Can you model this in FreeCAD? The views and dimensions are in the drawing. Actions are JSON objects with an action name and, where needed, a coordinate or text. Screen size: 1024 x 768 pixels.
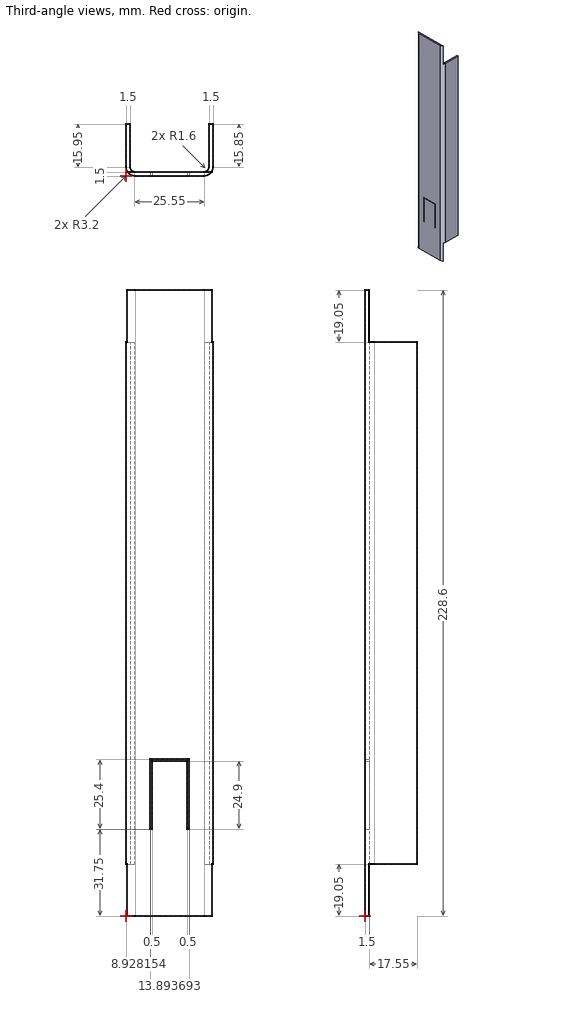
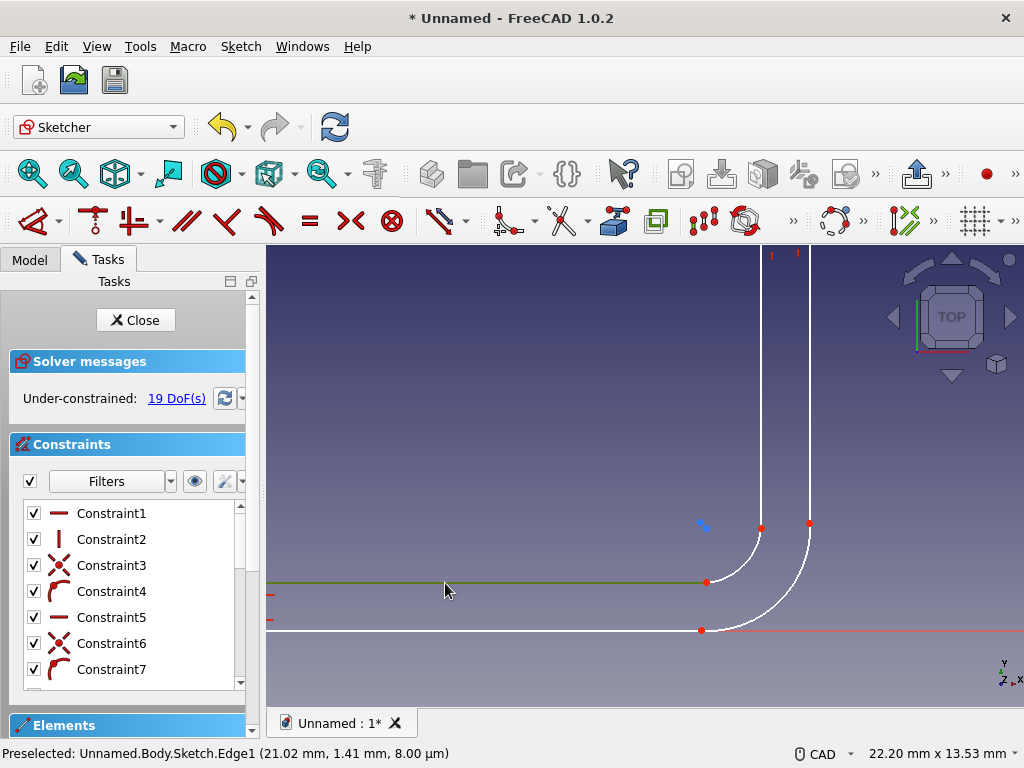
{"action": "scroll", "coordinate": [755, 575], "scroll_direction": "down", "scroll_amount": 5}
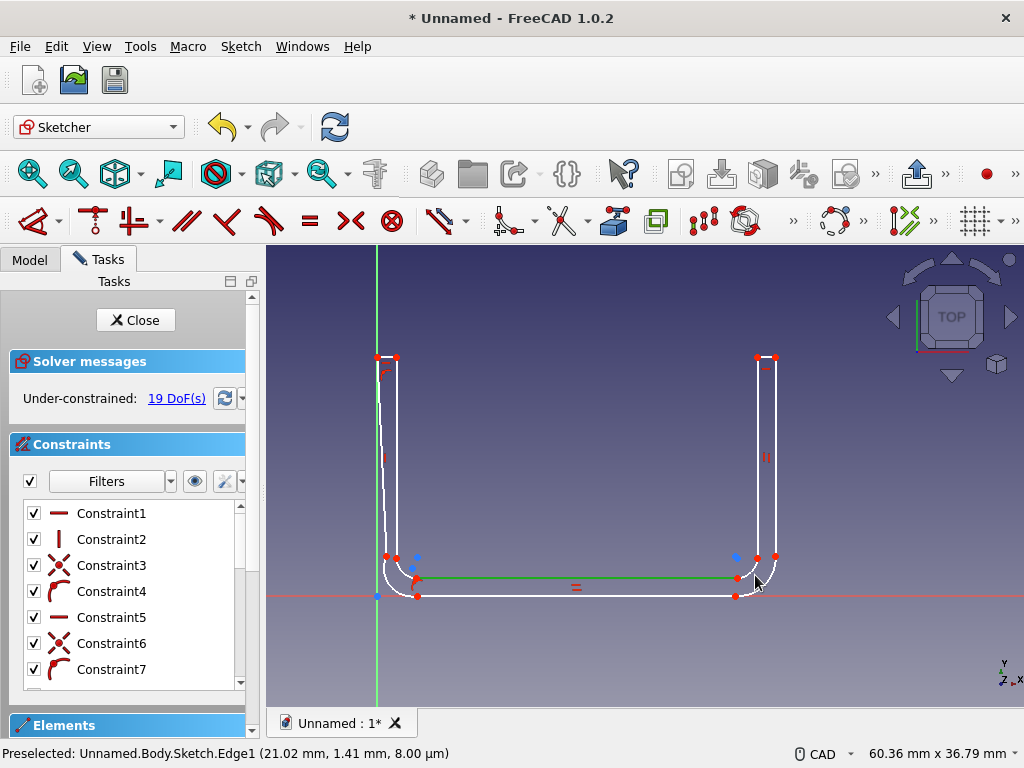
{"action": "scroll", "coordinate": [399, 567], "scroll_direction": "up", "scroll_amount": 2}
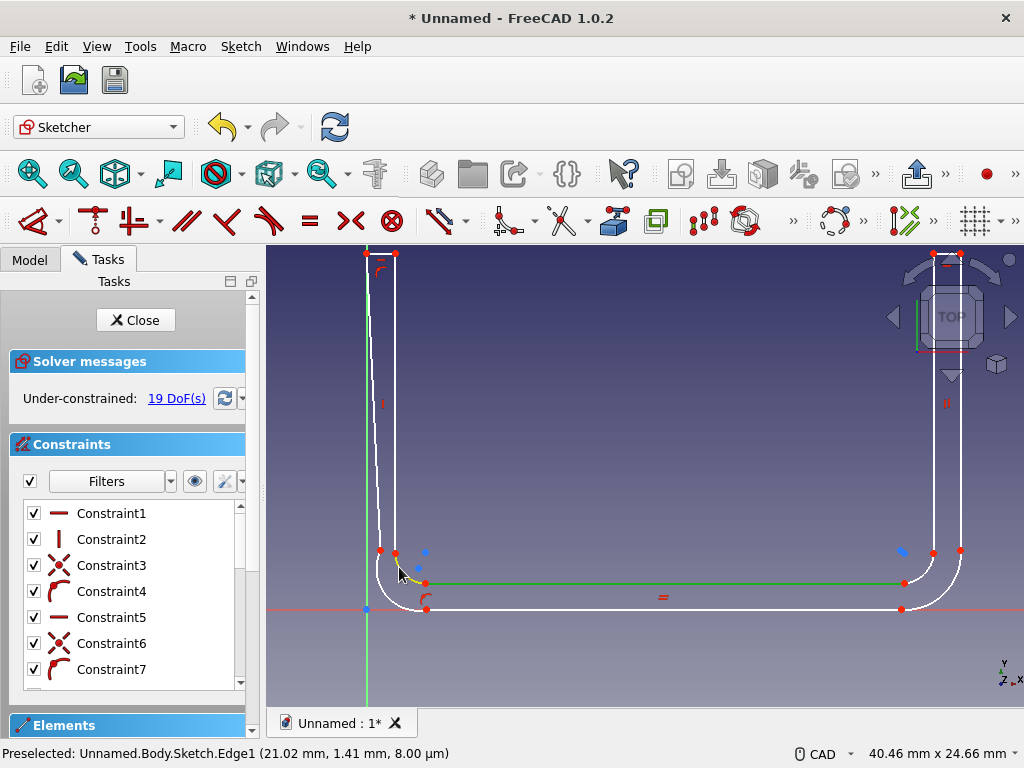
{"action": "left_click", "coordinate": [399, 567]}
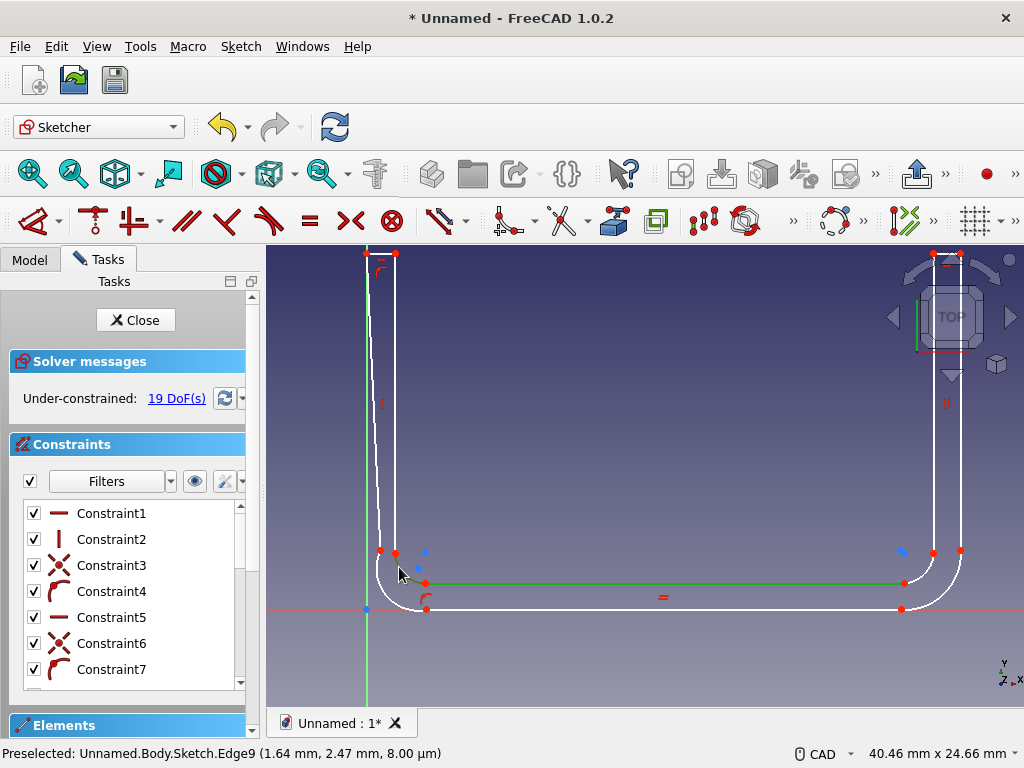
{"action": "left_click", "coordinate": [269, 222]}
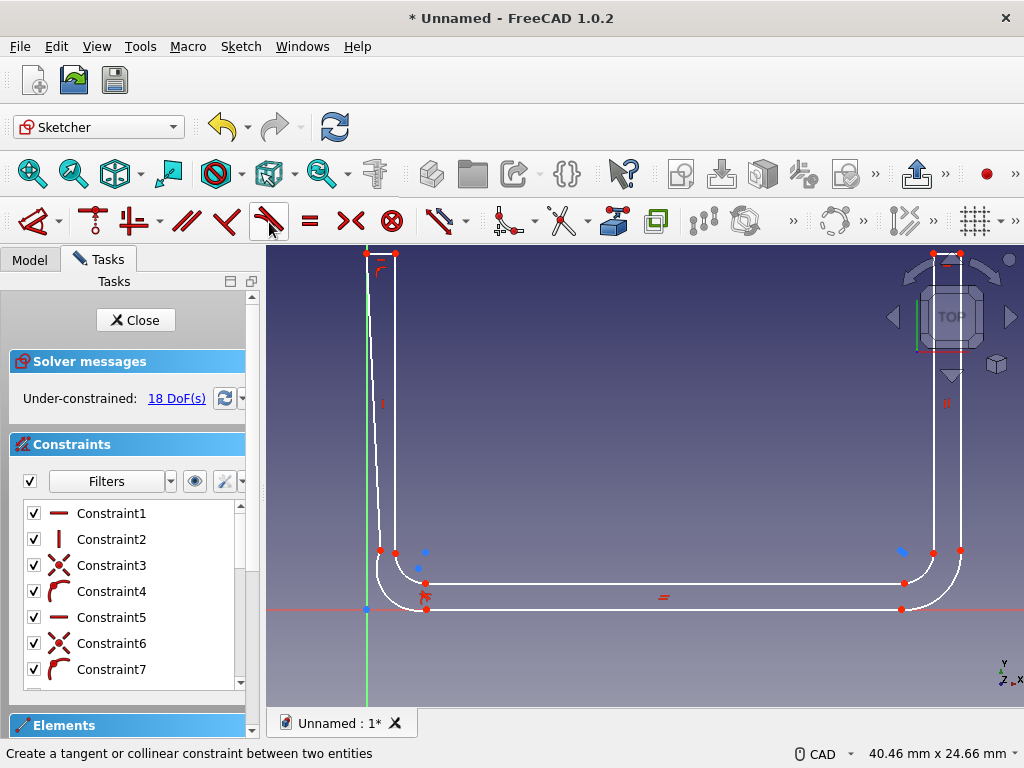
{"action": "left_click", "coordinate": [761, 584]}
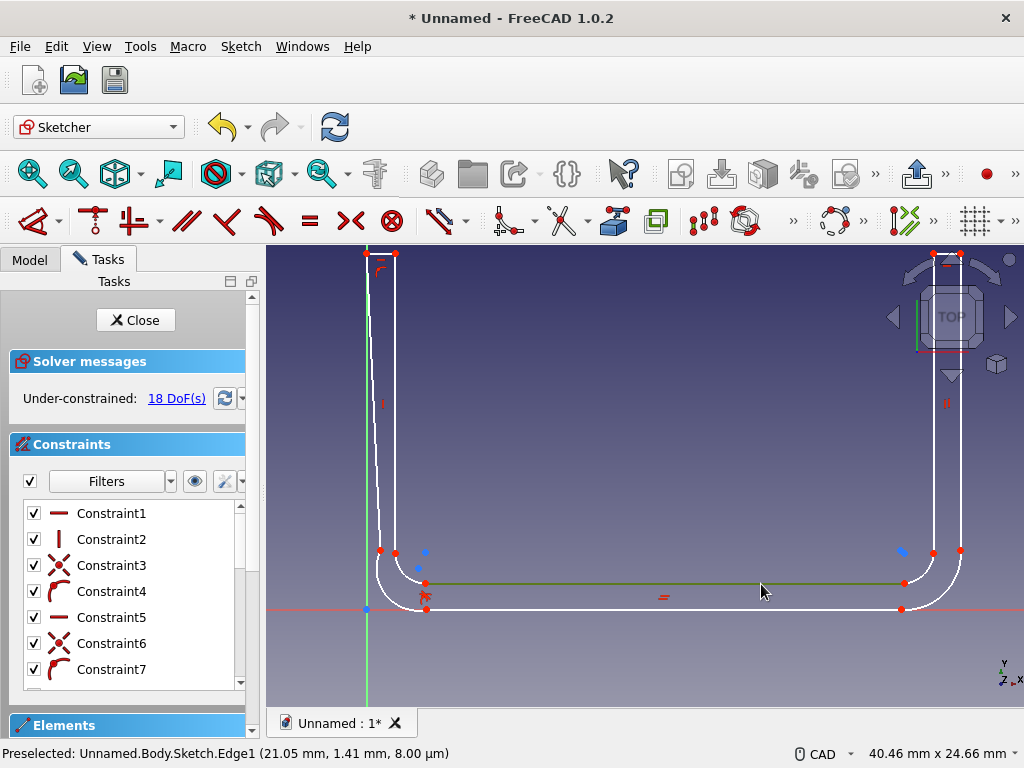
{"action": "scroll", "coordinate": [398, 566], "scroll_direction": "down", "scroll_amount": 2}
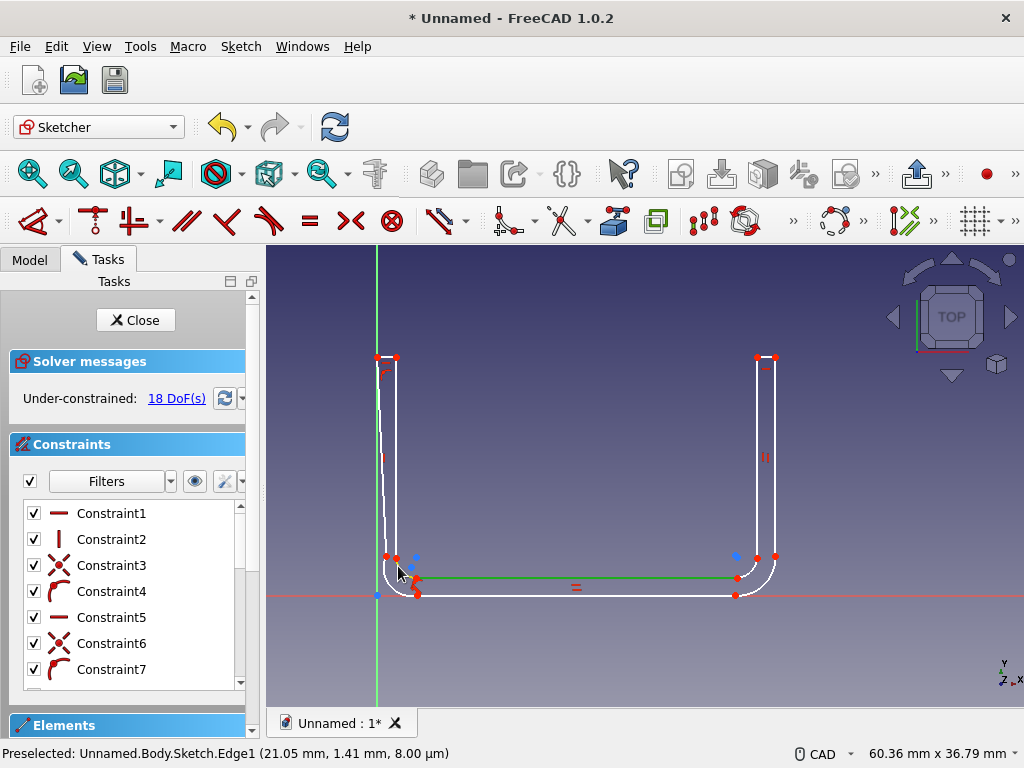
{"action": "scroll", "coordinate": [746, 575], "scroll_direction": "up", "scroll_amount": 3}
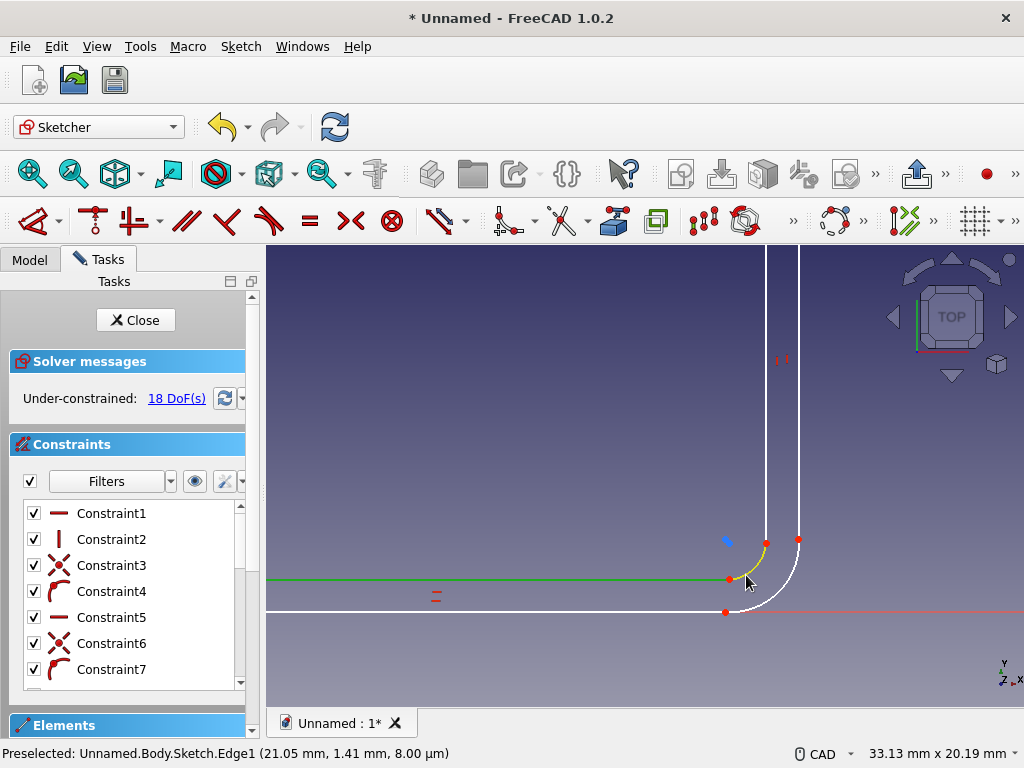
{"action": "left_click", "coordinate": [745, 575]}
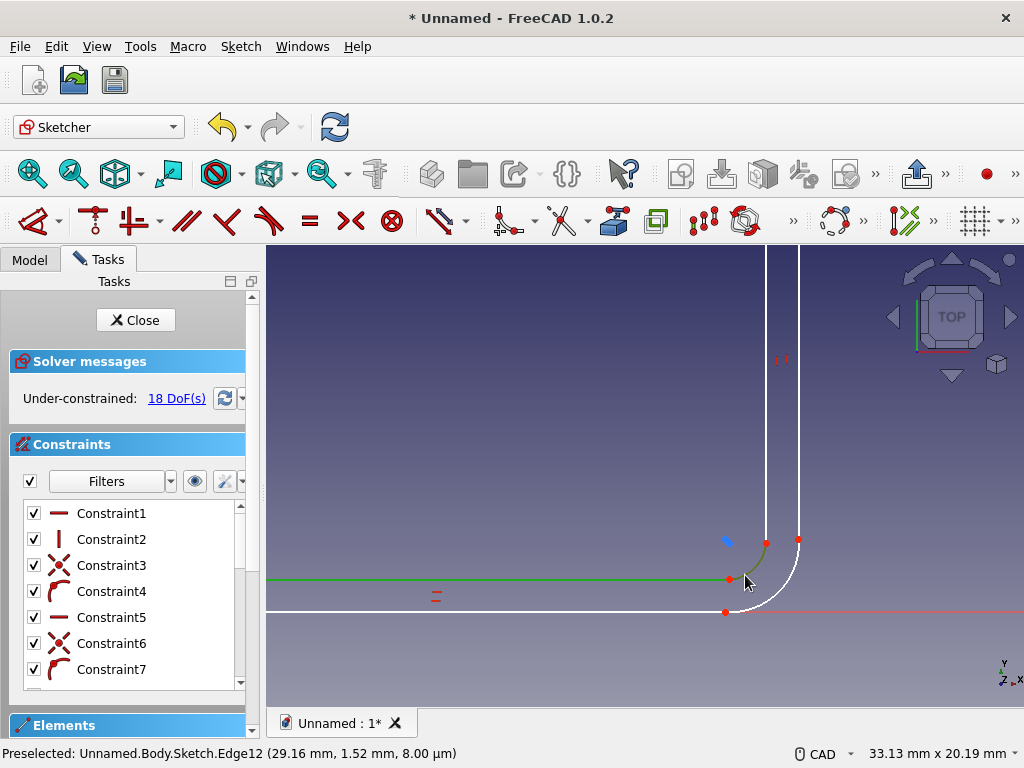
{"action": "left_click", "coordinate": [269, 222]}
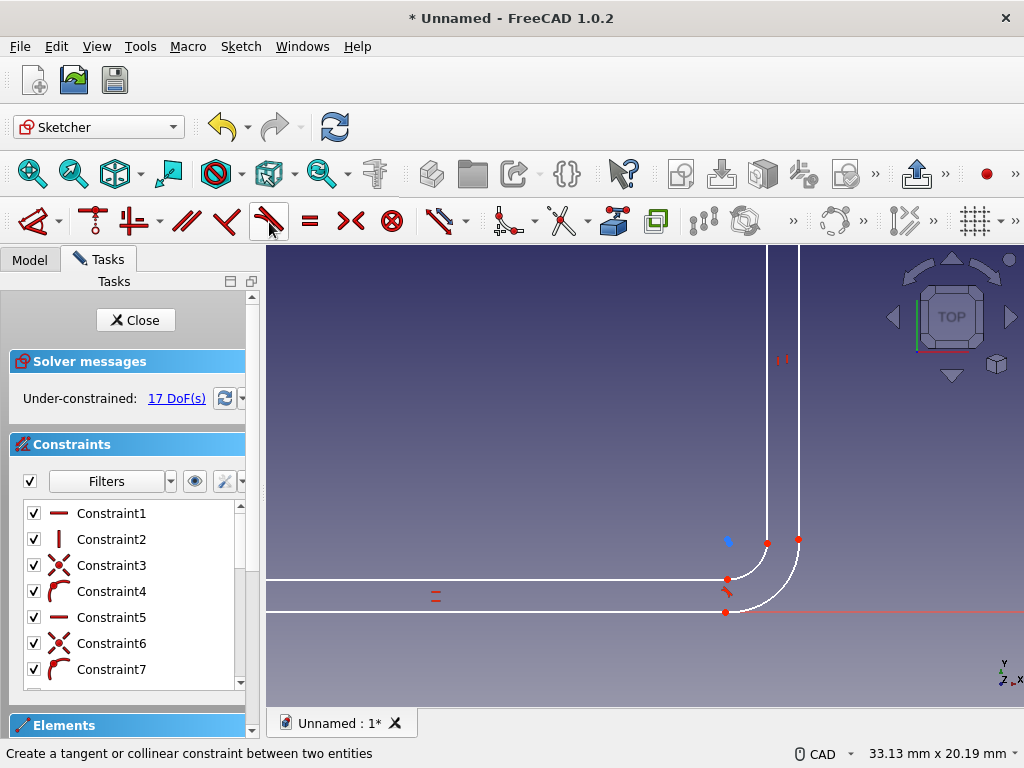
{"action": "scroll", "coordinate": [747, 576], "scroll_direction": "down", "scroll_amount": 3}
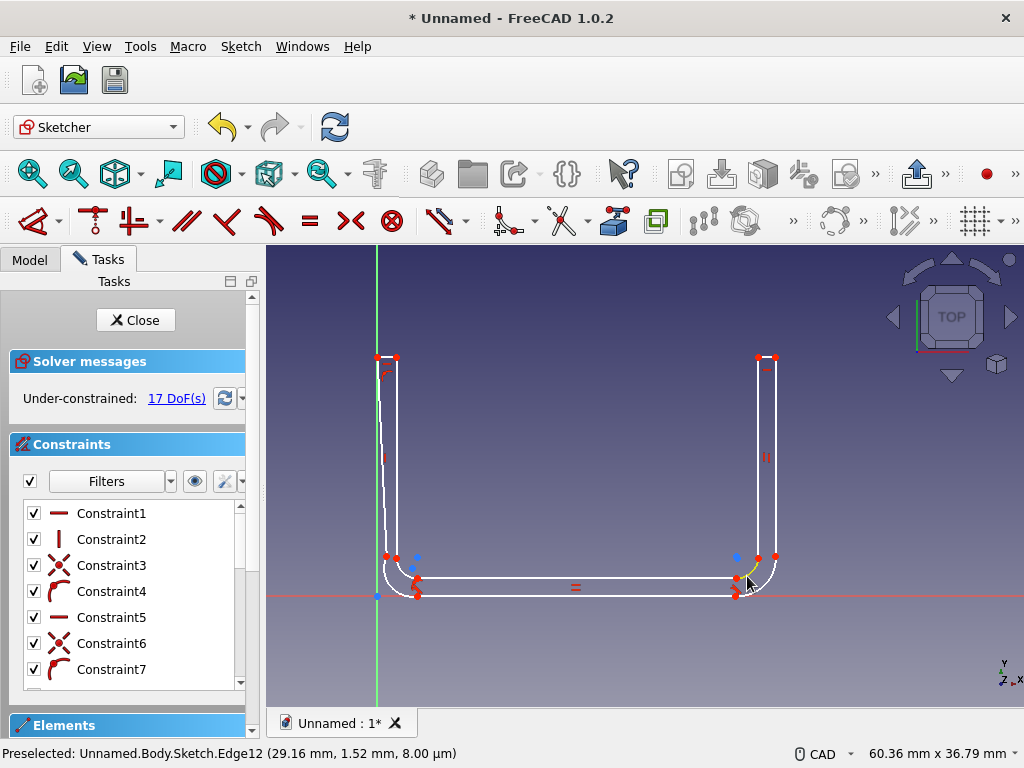
{"action": "left_click", "coordinate": [397, 498]}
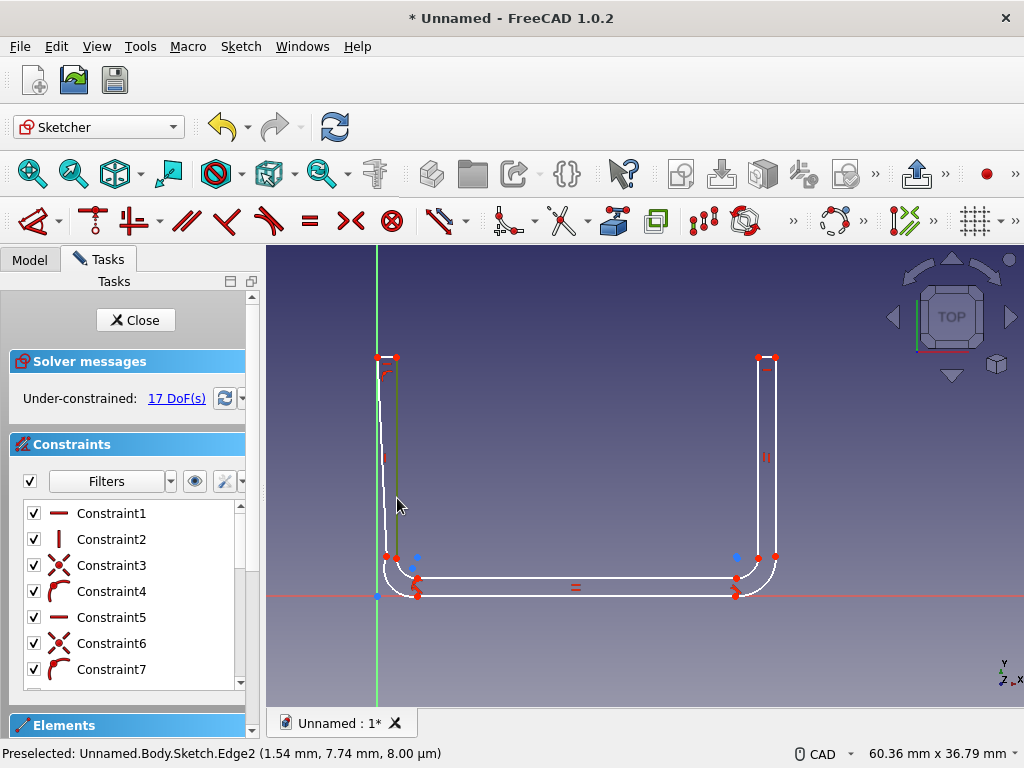
{"action": "scroll", "coordinate": [399, 568], "scroll_direction": "up", "scroll_amount": 2}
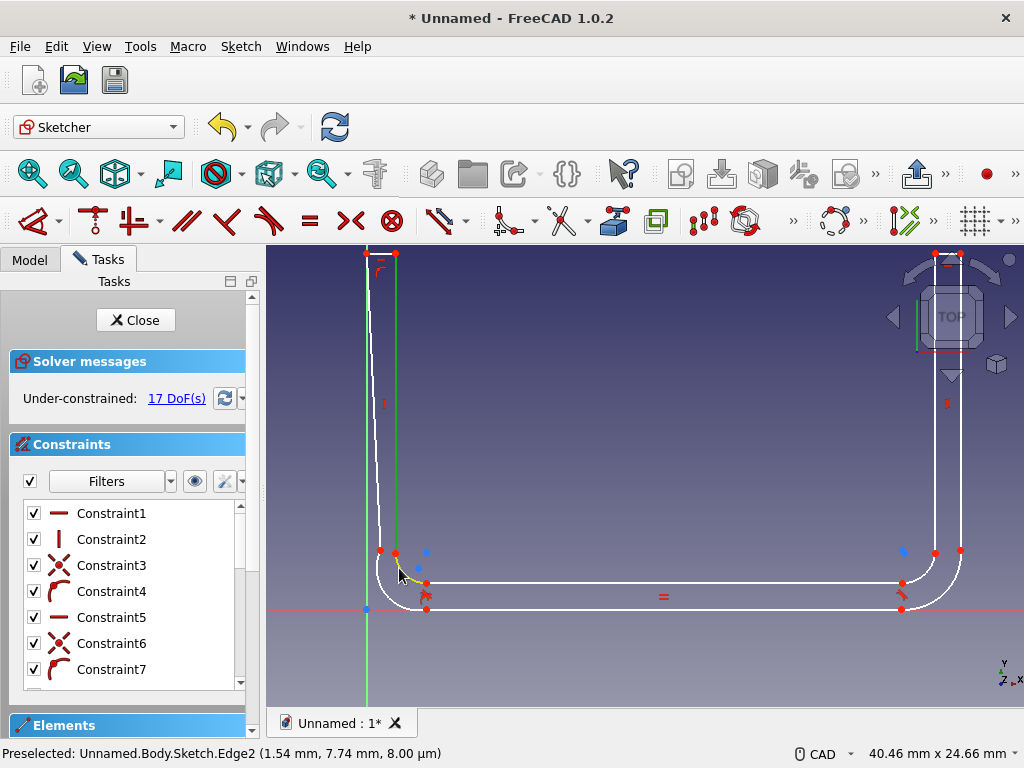
{"action": "left_click", "coordinate": [399, 567]}